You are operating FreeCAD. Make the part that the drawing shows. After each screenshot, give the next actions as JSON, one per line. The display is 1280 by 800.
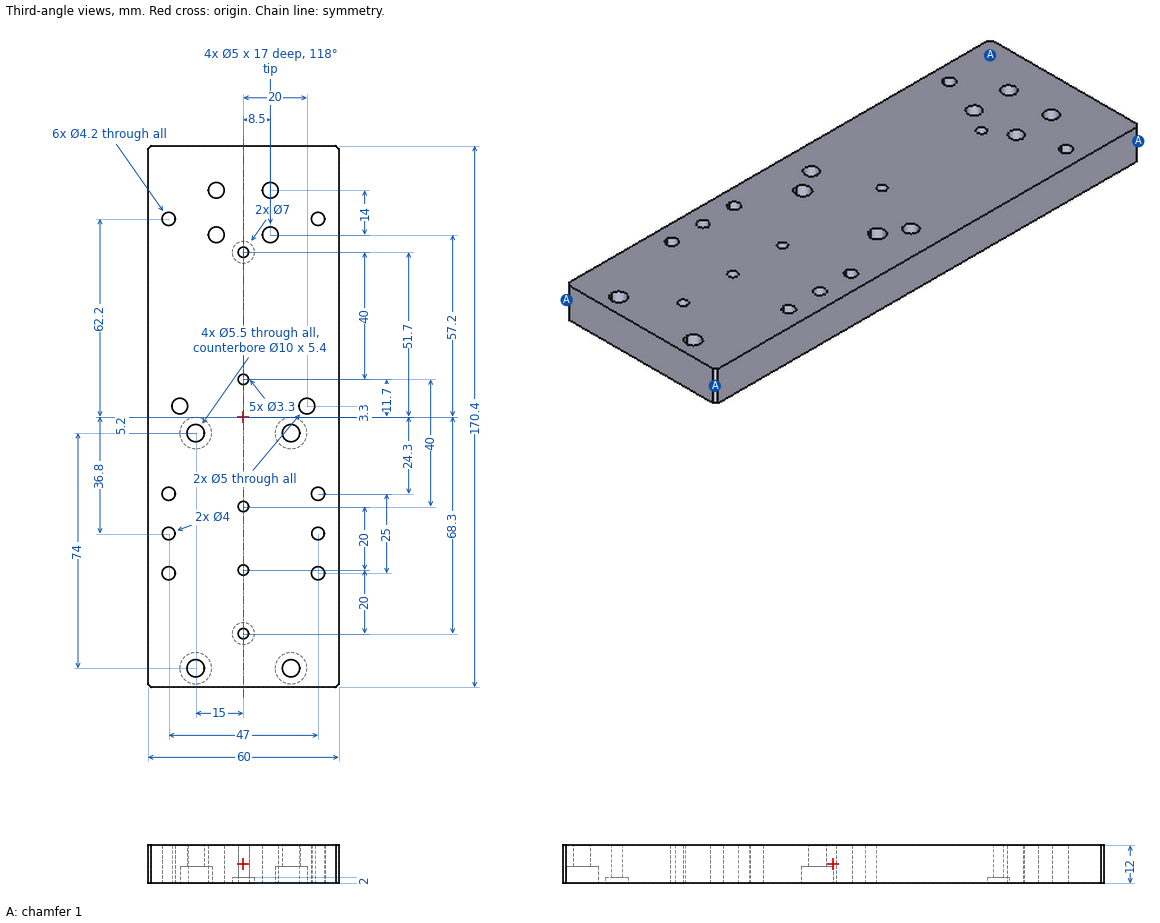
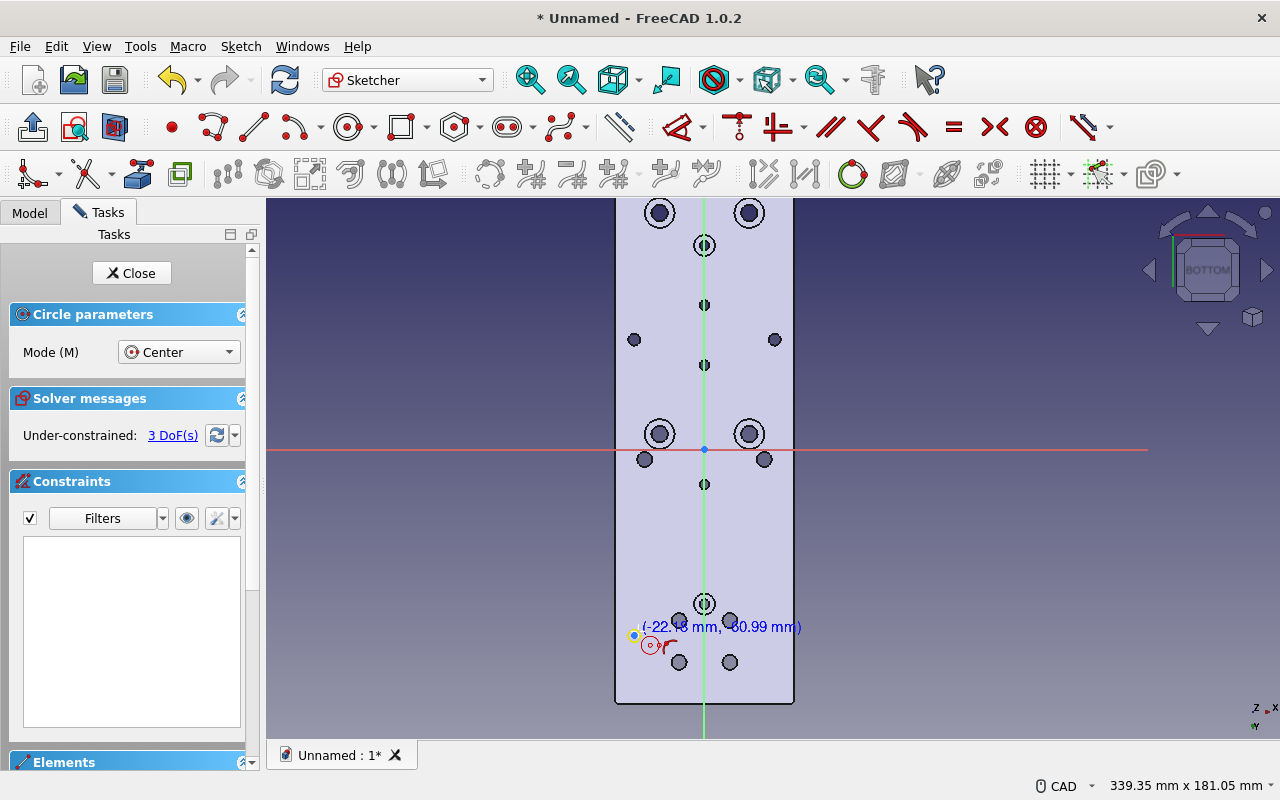
{"action": "scroll", "coordinate": [775, 377], "scroll_direction": "up", "scroll_amount": 7}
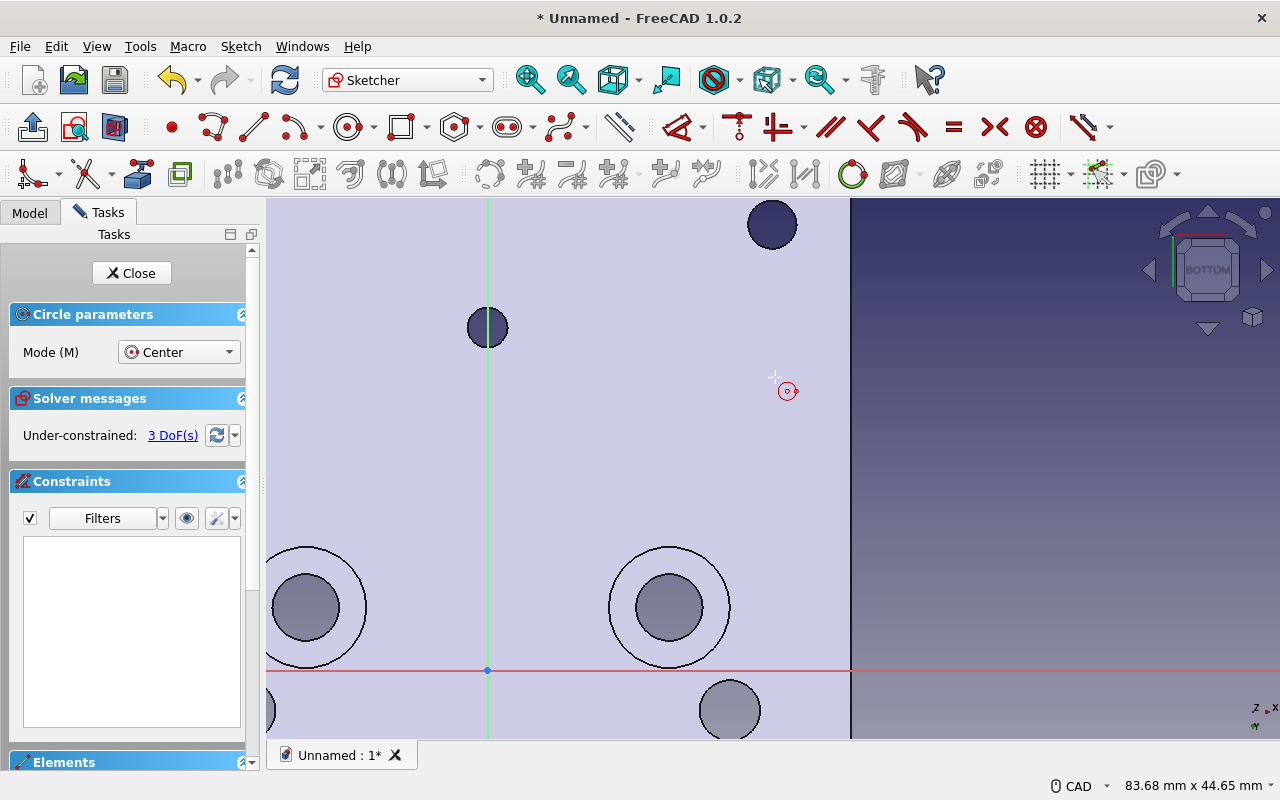
{"action": "scroll", "coordinate": [776, 377], "scroll_direction": "down", "scroll_amount": 7}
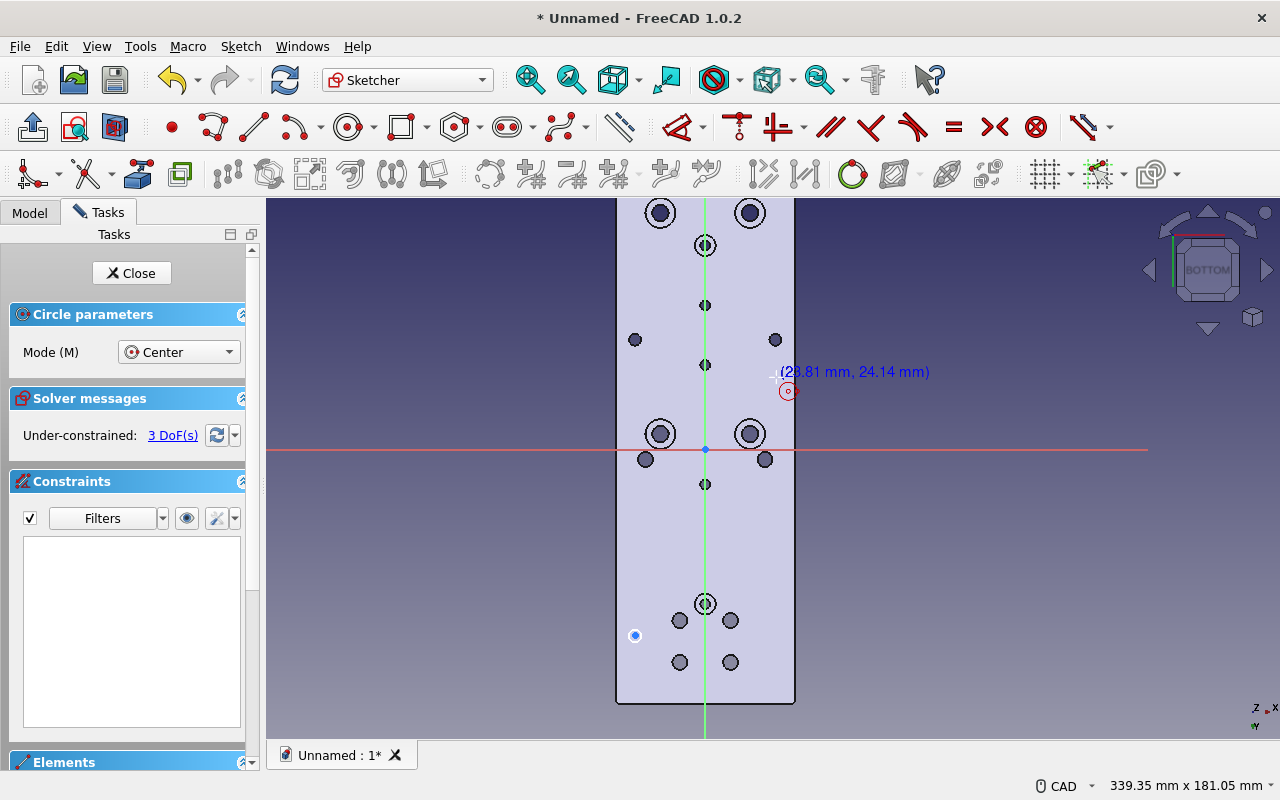
{"action": "left_click", "coordinate": [775, 377]}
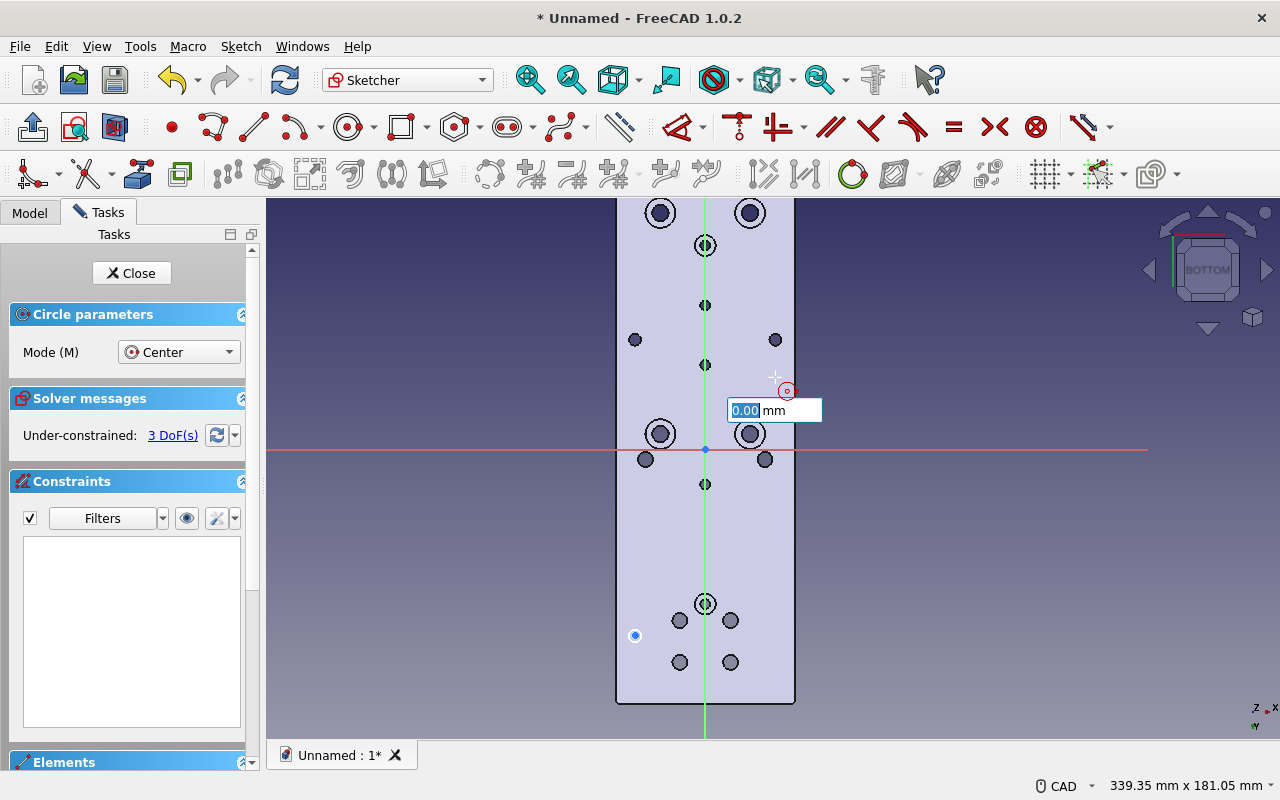
{"action": "scroll", "coordinate": [780, 373], "scroll_direction": "up", "scroll_amount": 5}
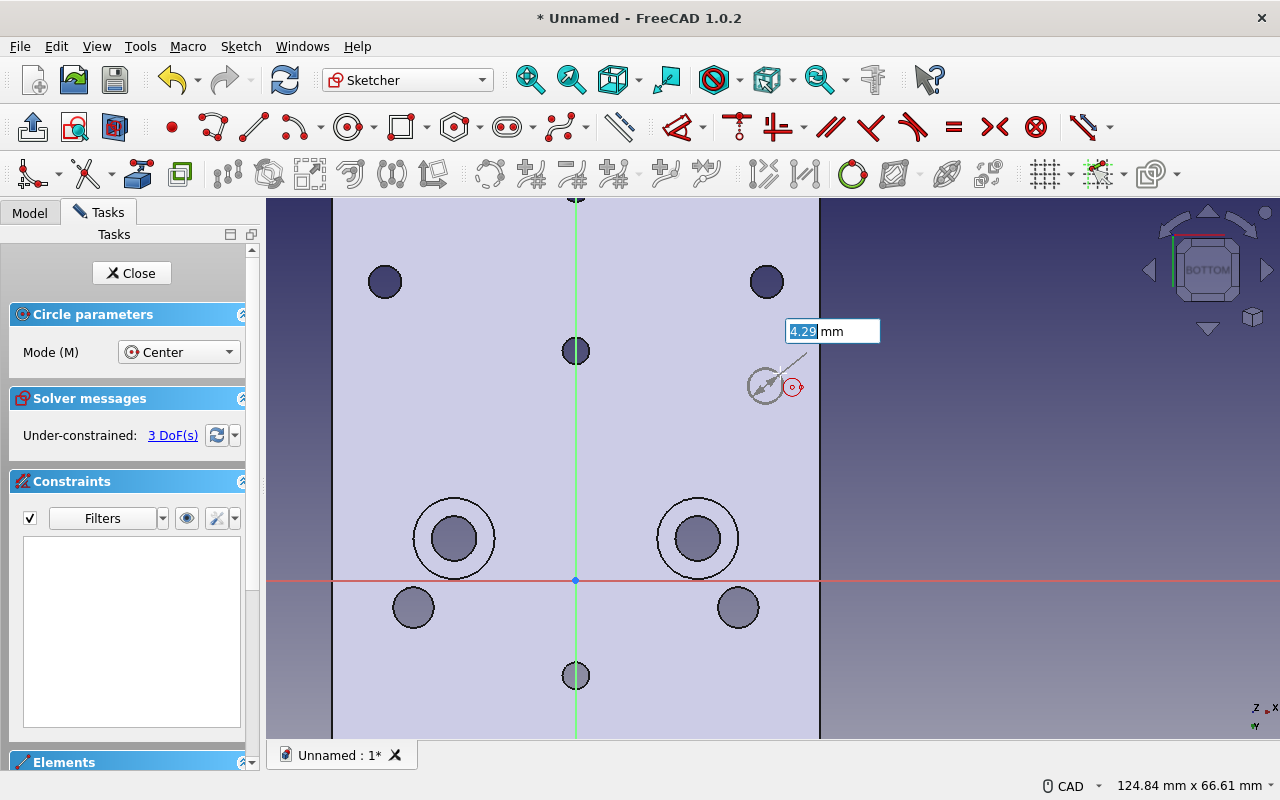
{"action": "left_click", "coordinate": [779, 371]}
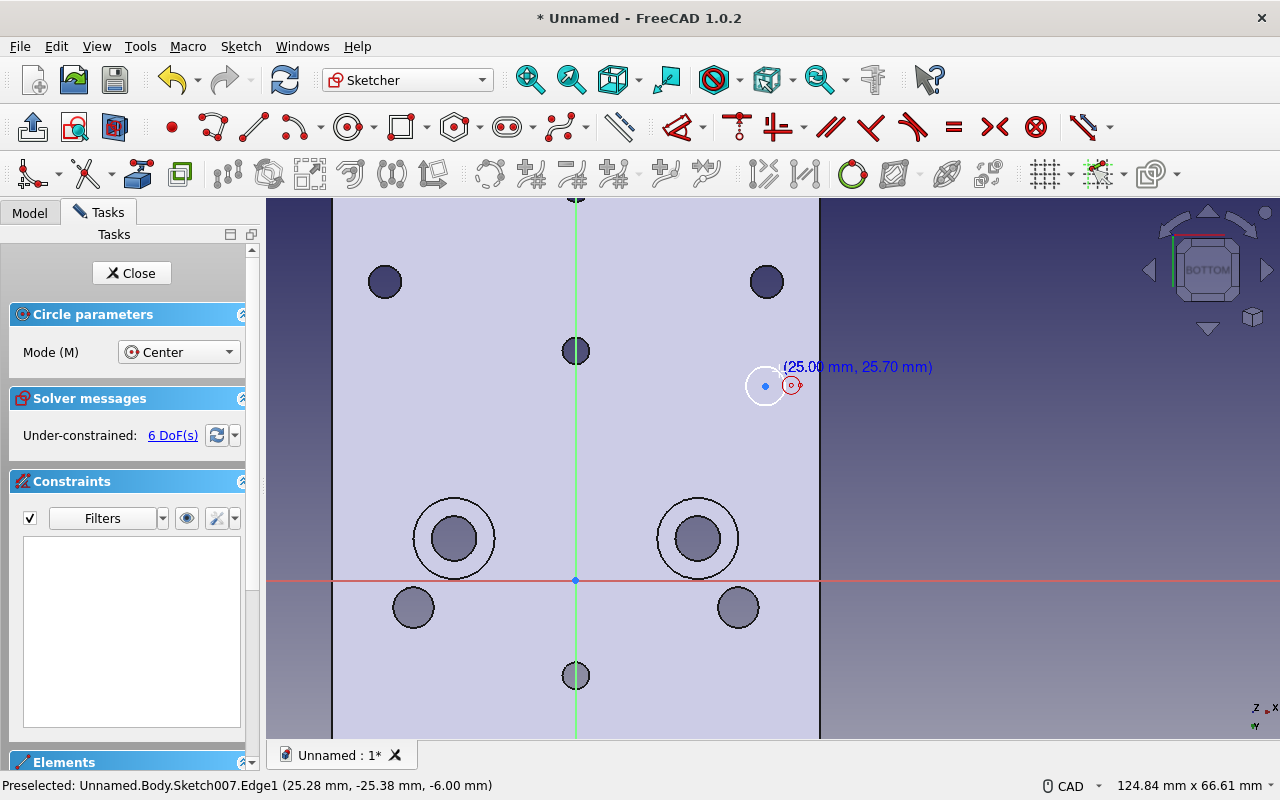
{"action": "scroll", "coordinate": [779, 373], "scroll_direction": "down", "scroll_amount": 5}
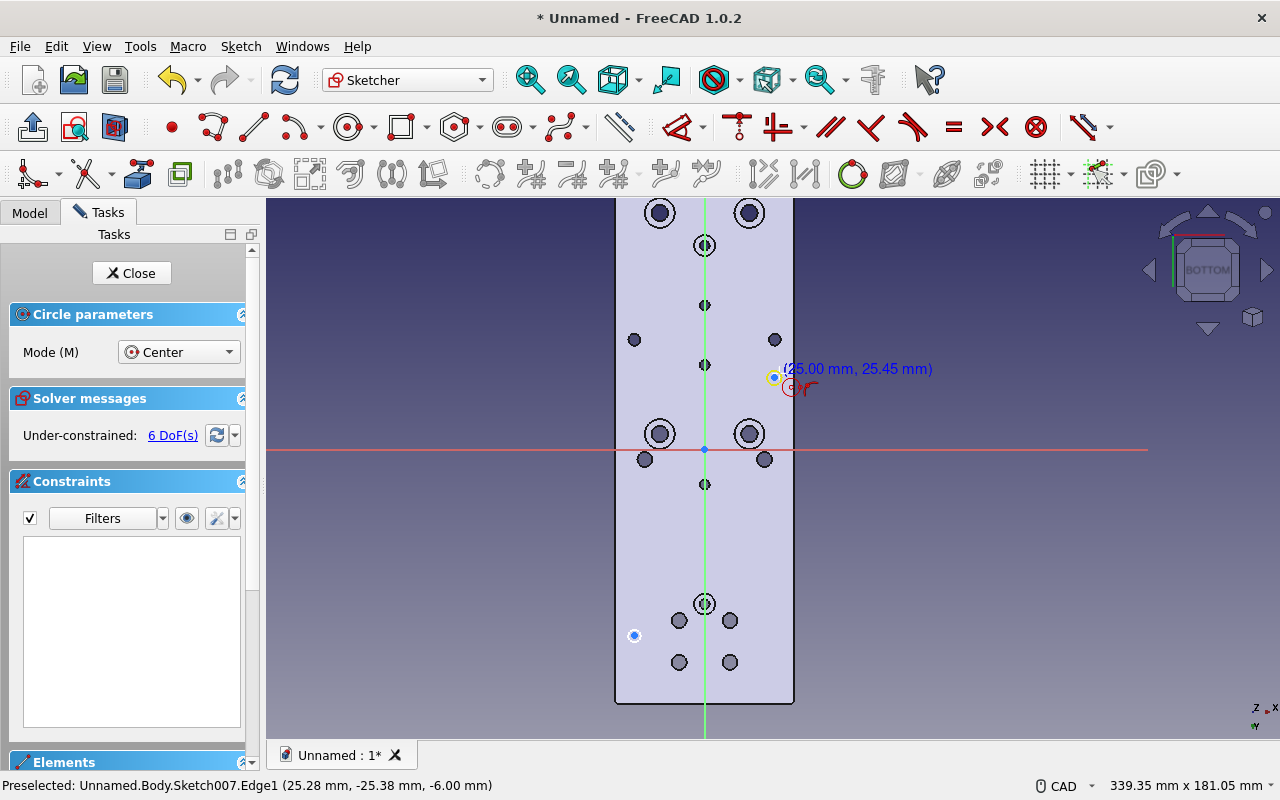
{"action": "scroll", "coordinate": [775, 302], "scroll_direction": "up", "scroll_amount": 7}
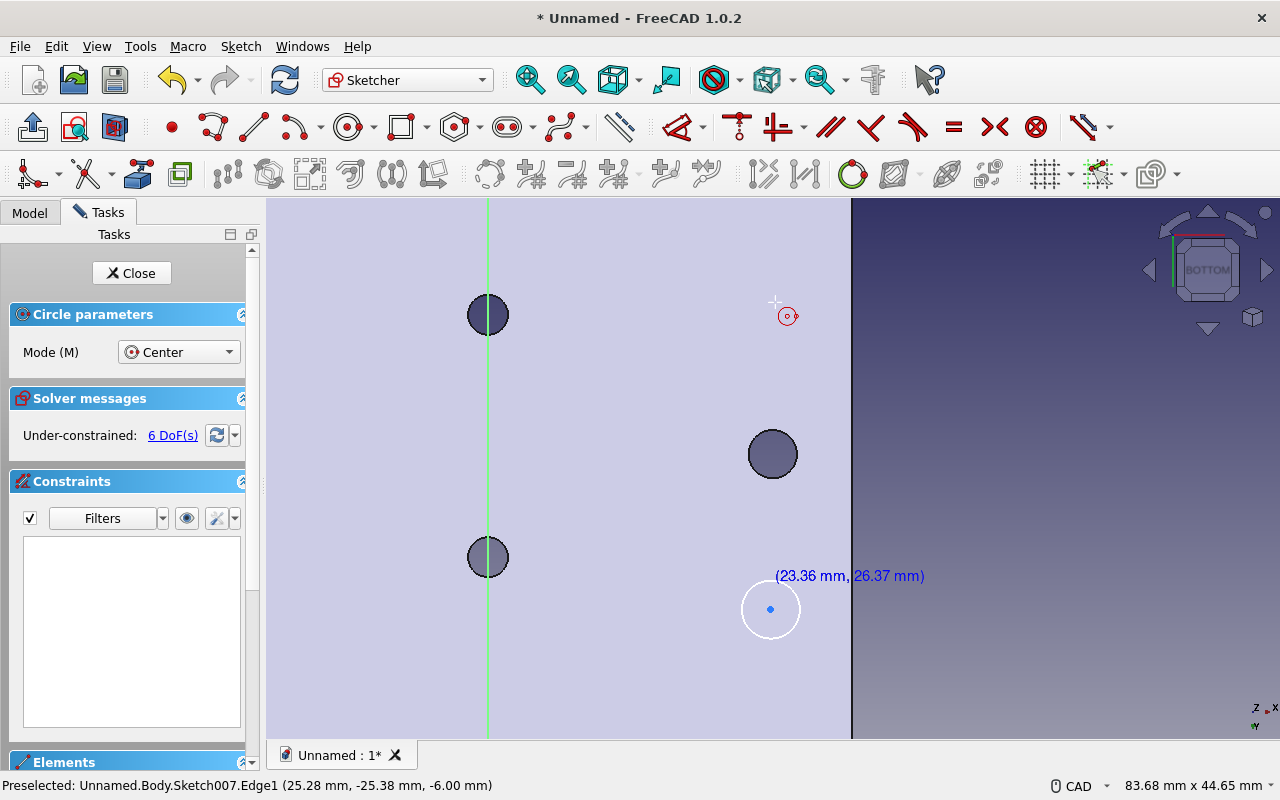
{"action": "scroll", "coordinate": [775, 302], "scroll_direction": "down", "scroll_amount": 7}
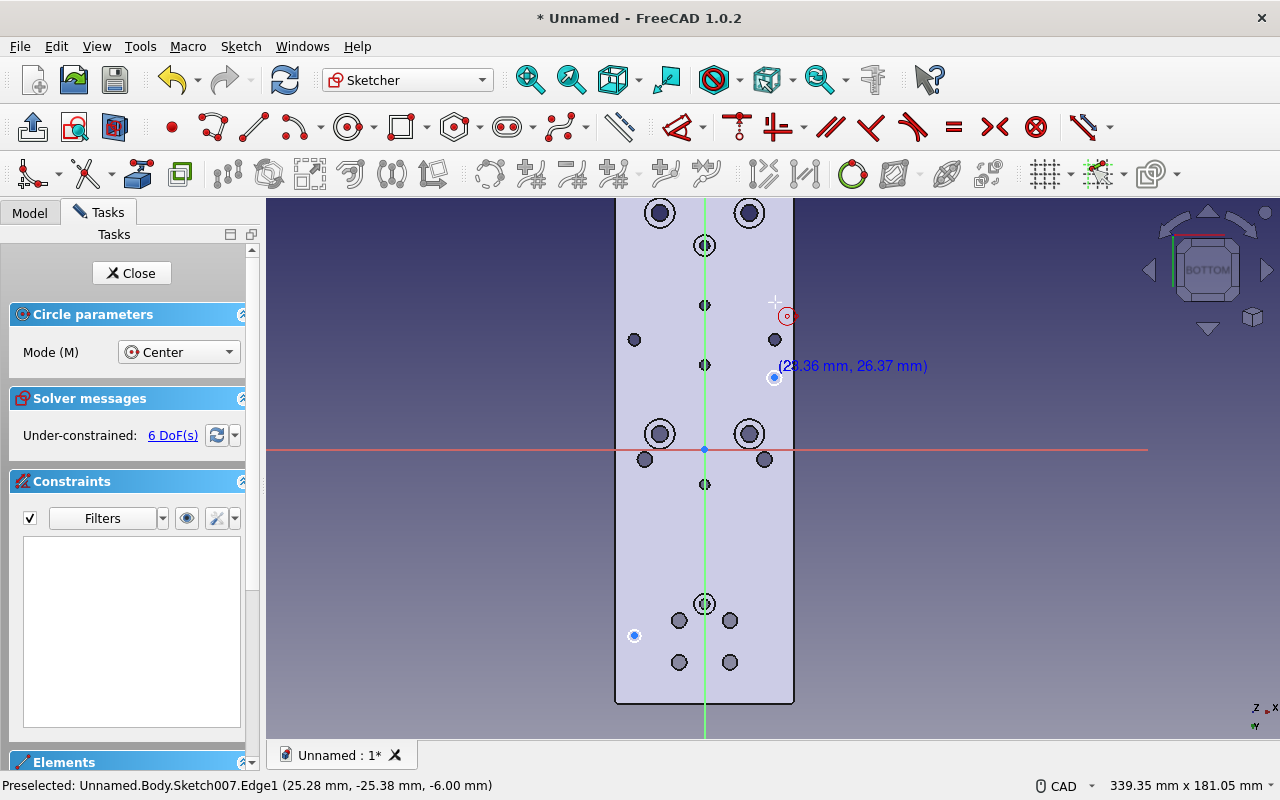
{"action": "left_click", "coordinate": [775, 302]}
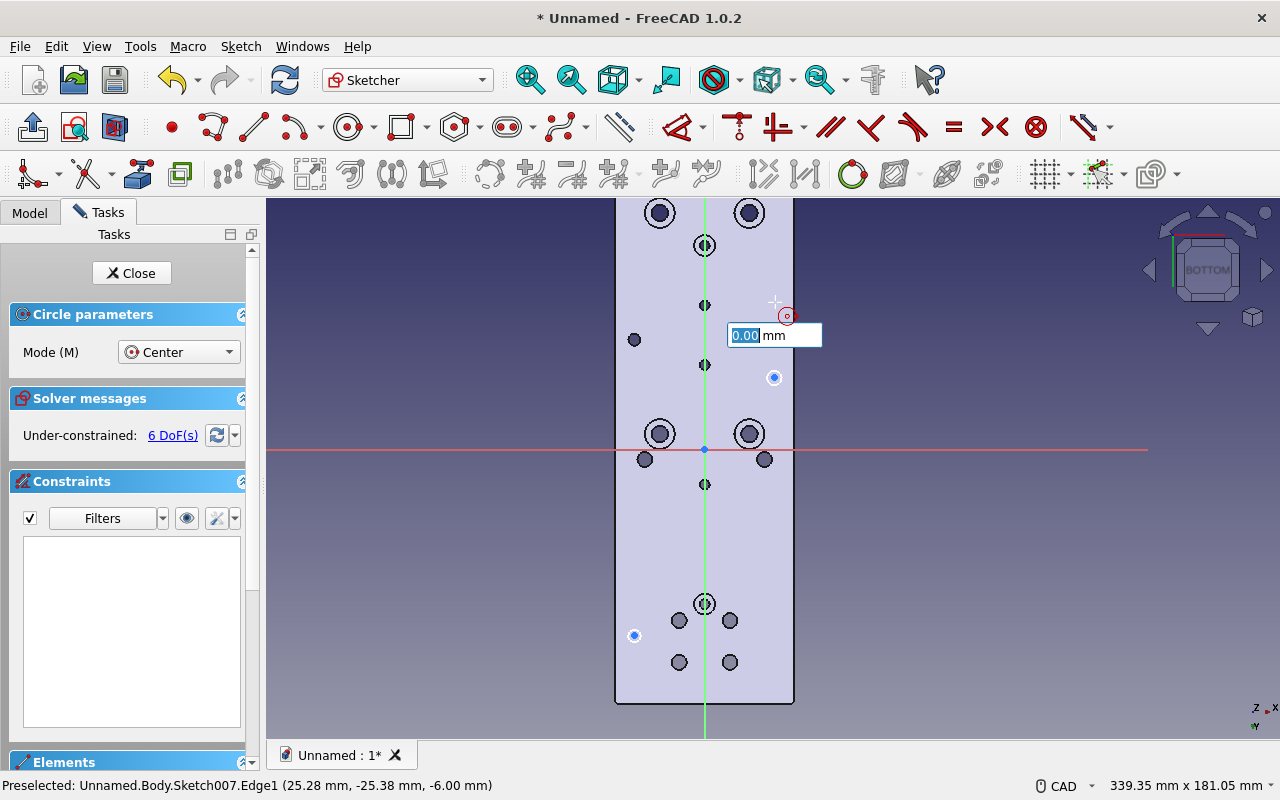
{"action": "scroll", "coordinate": [779, 298], "scroll_direction": "up", "scroll_amount": 5}